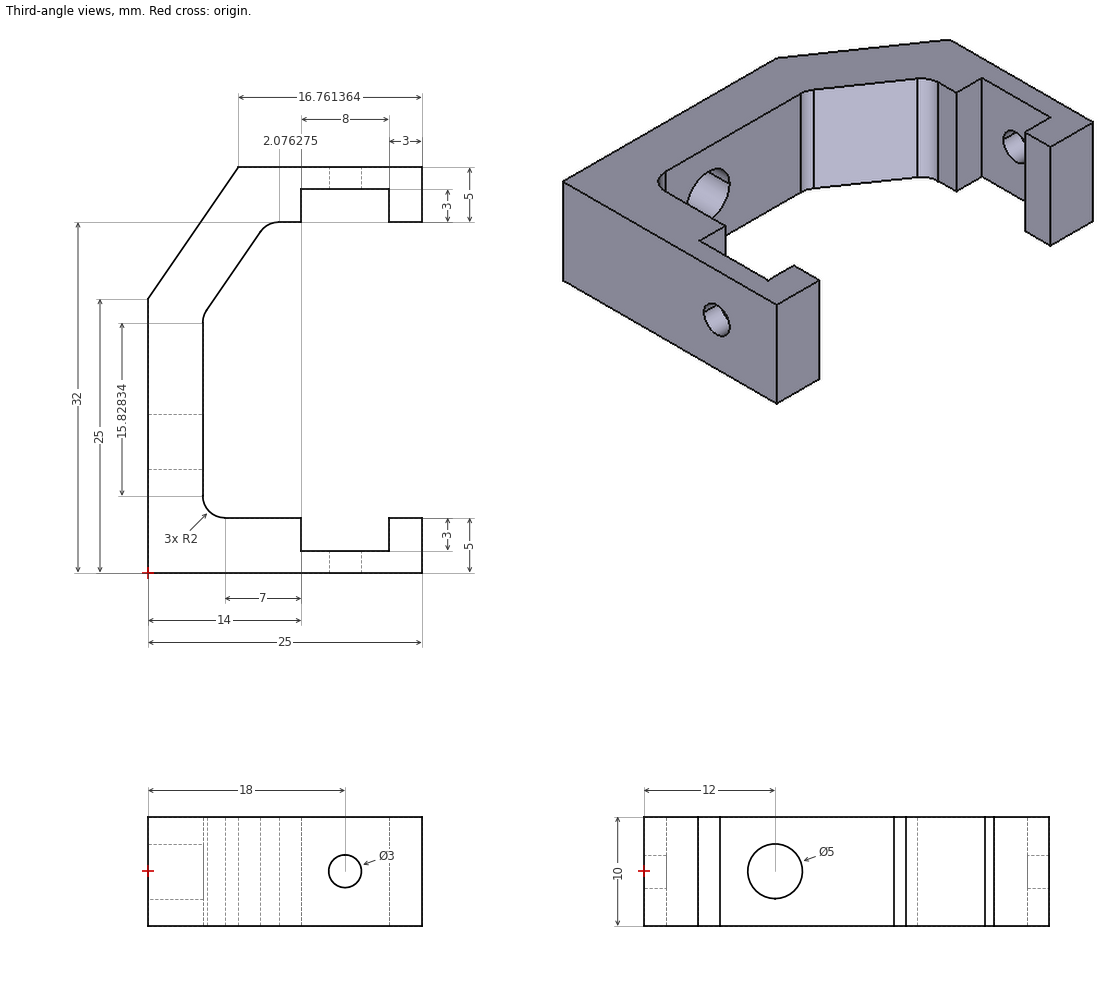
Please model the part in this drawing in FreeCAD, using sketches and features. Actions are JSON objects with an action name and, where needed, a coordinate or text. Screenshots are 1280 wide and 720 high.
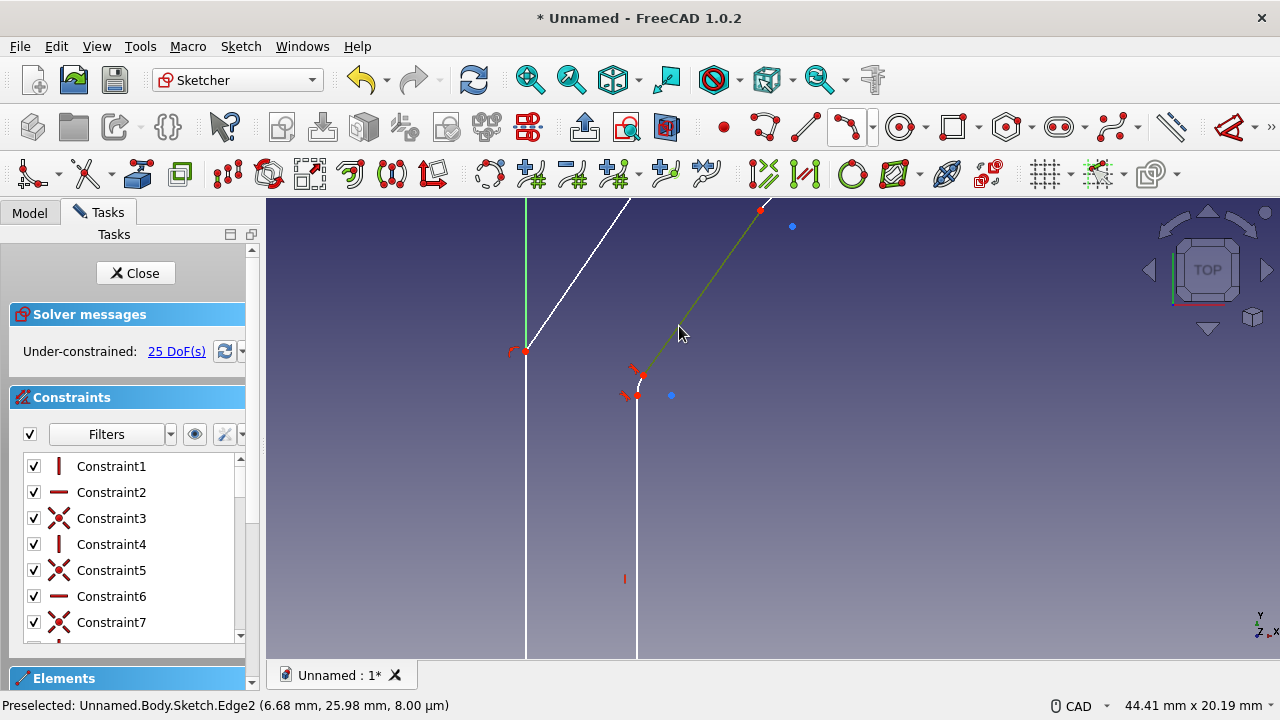
{"action": "scroll", "coordinate": [642, 388], "scroll_direction": "down", "scroll_amount": 5}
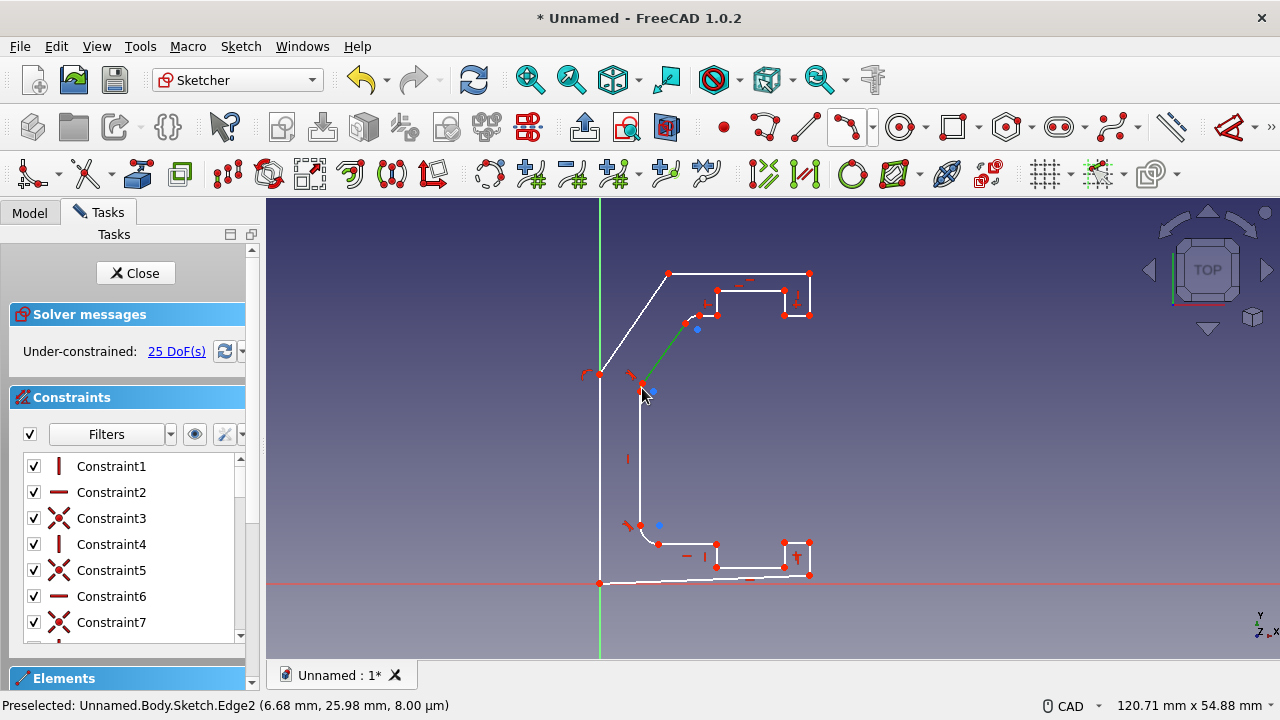
{"action": "scroll", "coordinate": [695, 316], "scroll_direction": "up", "scroll_amount": 6}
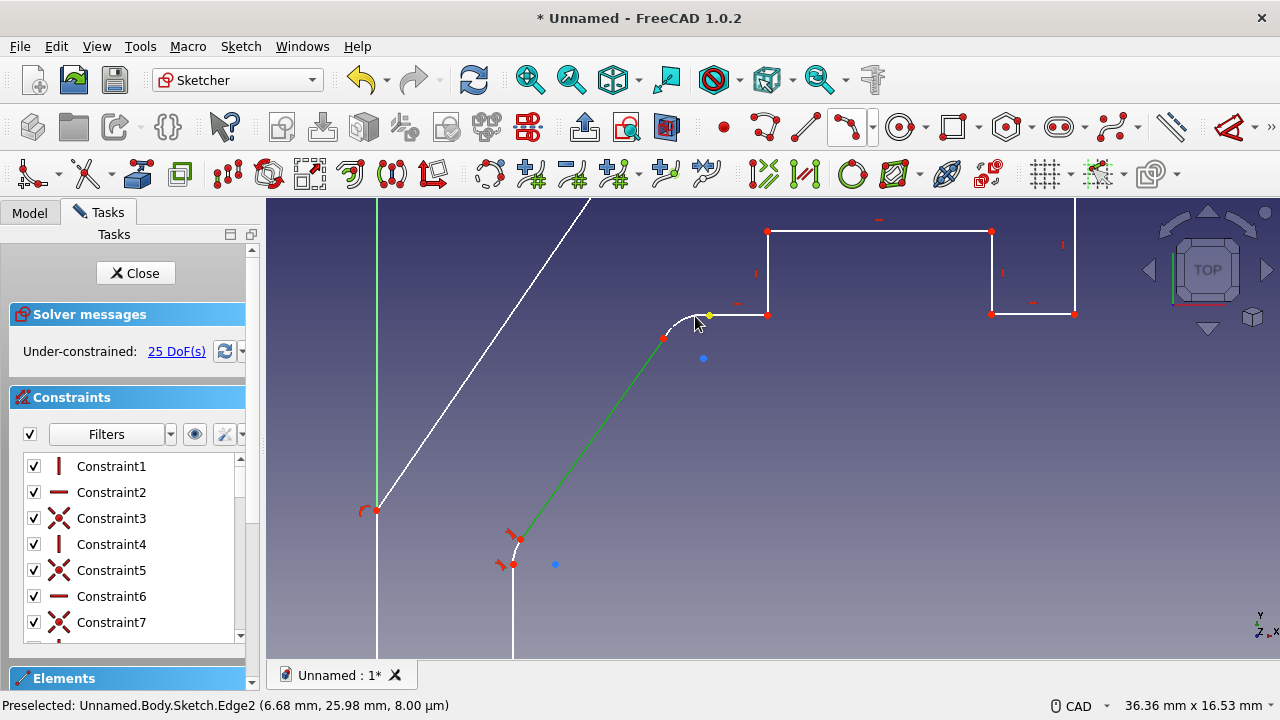
{"action": "left_click", "coordinate": [693, 316]}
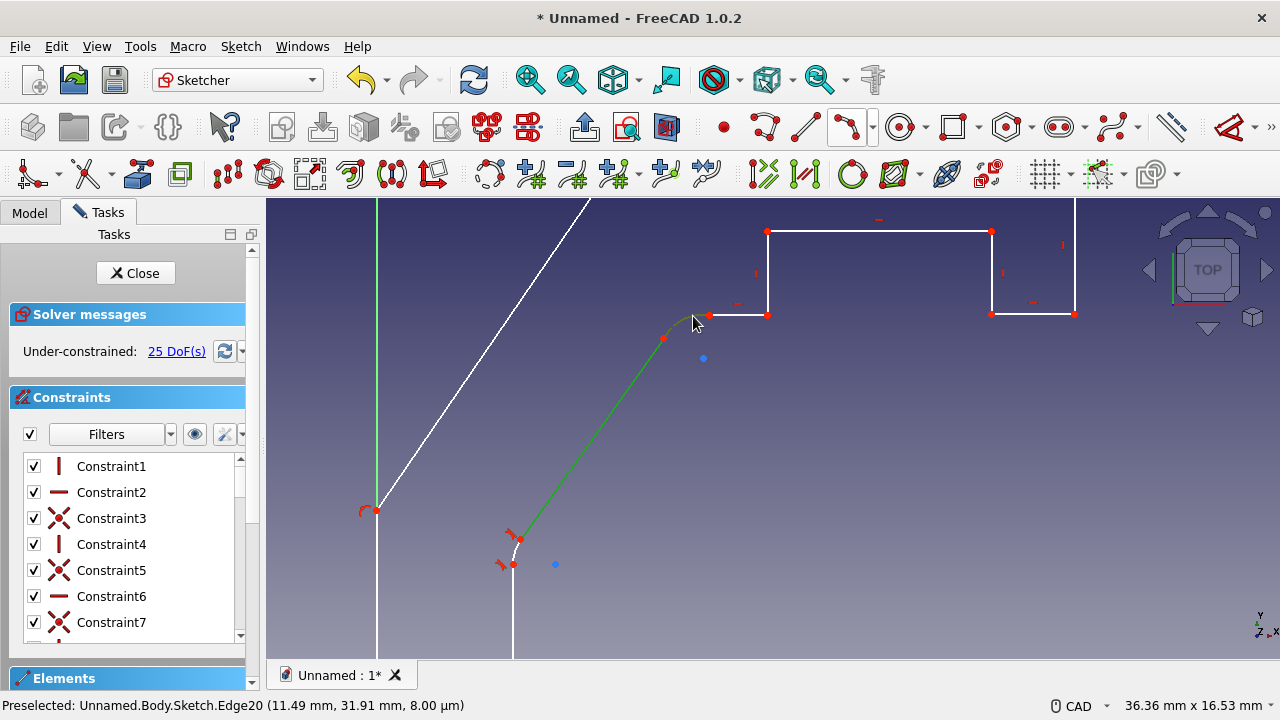
{"action": "key", "text": "t"}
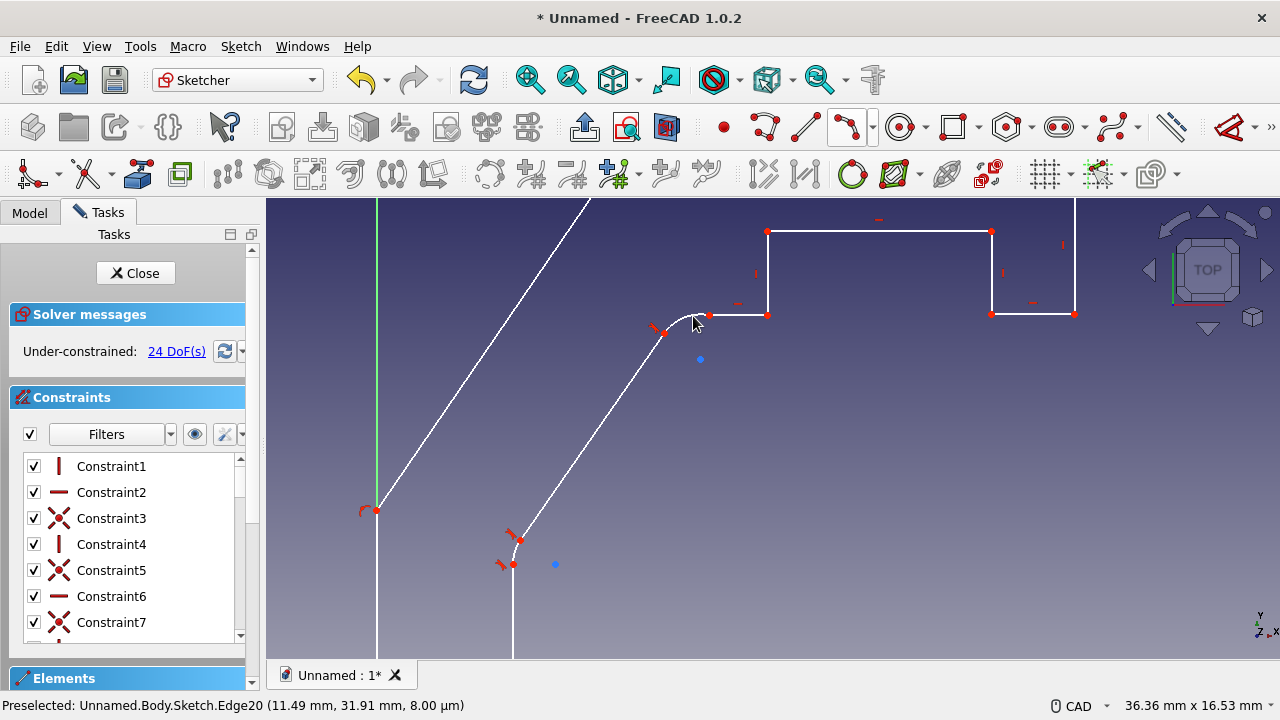
{"action": "left_click", "coordinate": [727, 315]}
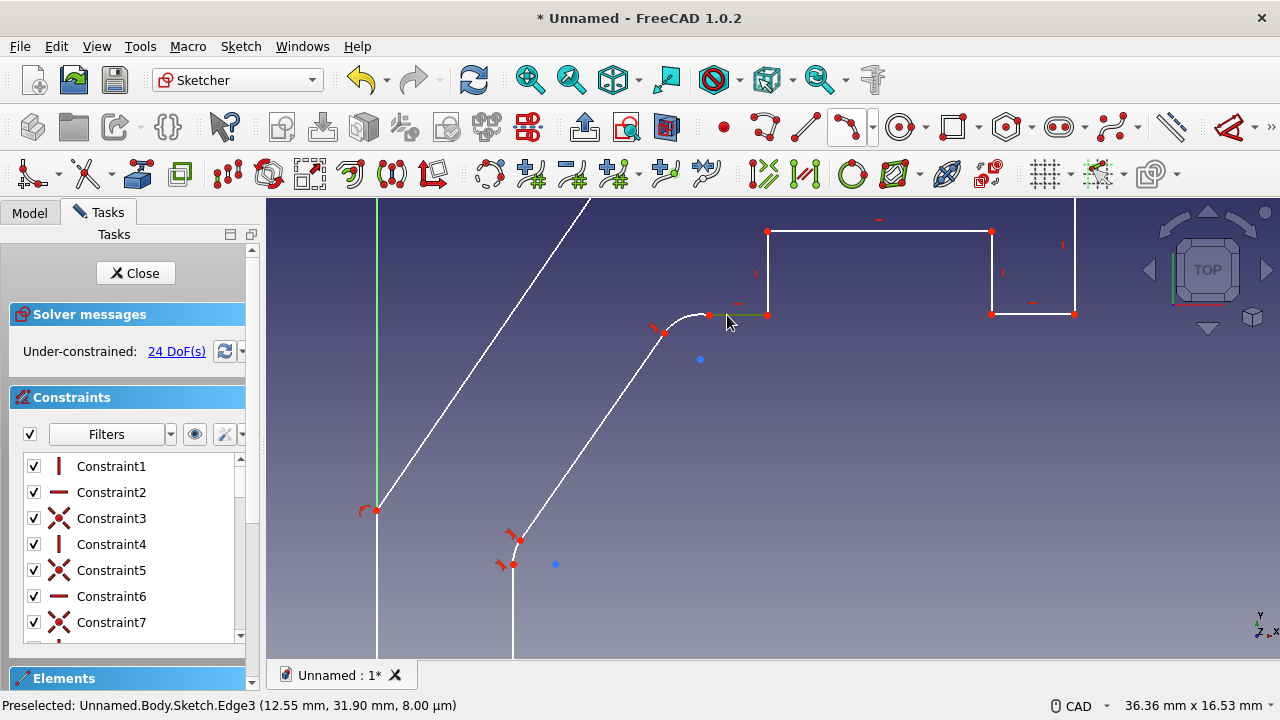
{"action": "left_click", "coordinate": [694, 315]}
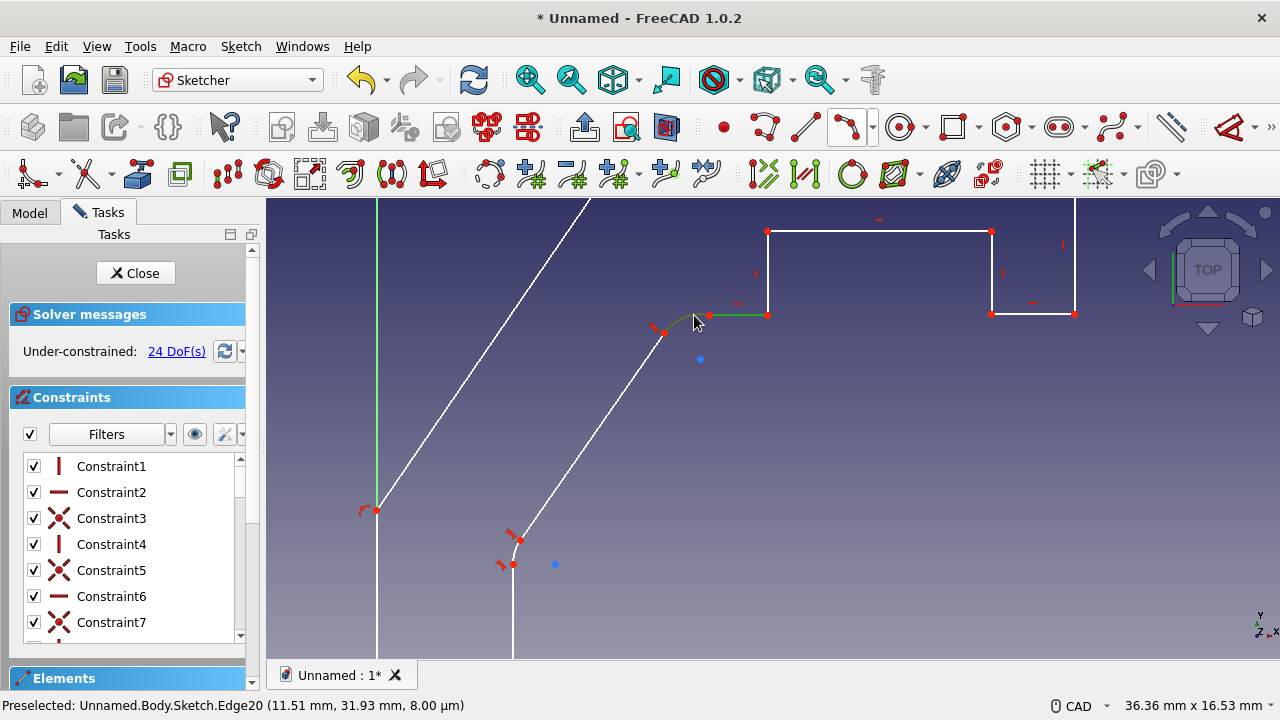
{"action": "key", "text": "t"}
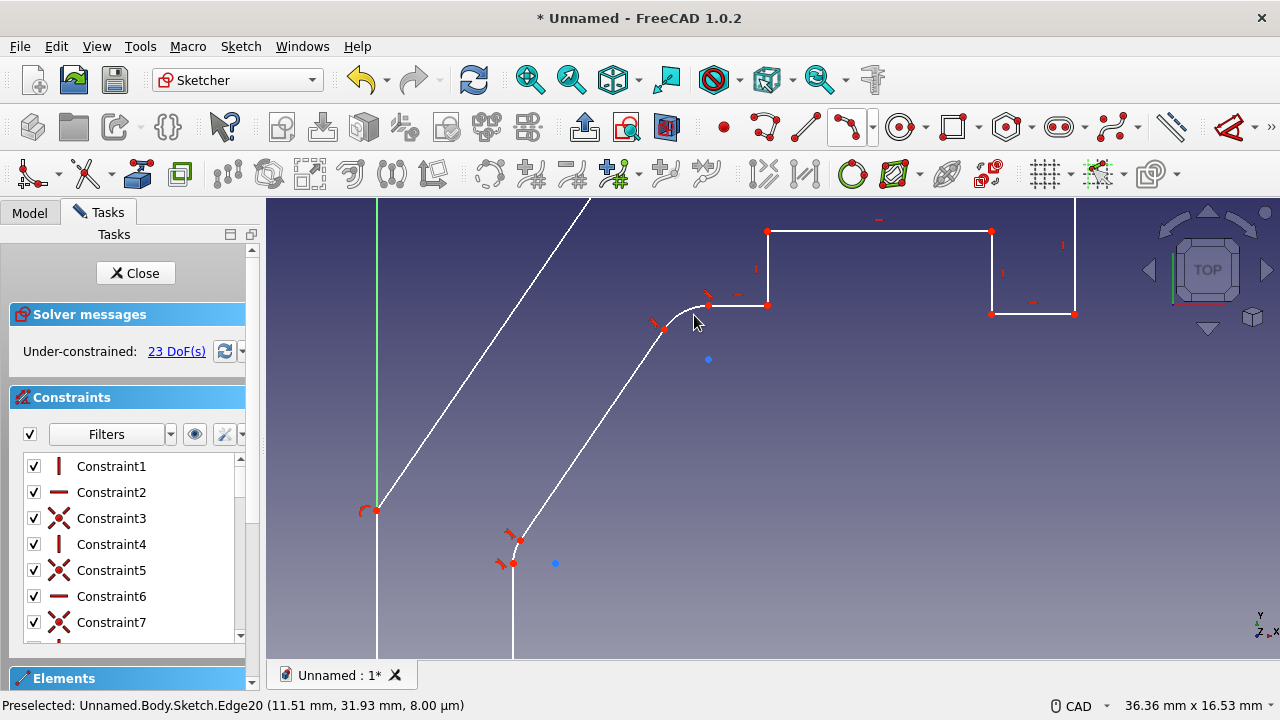
{"action": "scroll", "coordinate": [695, 316], "scroll_direction": "down", "scroll_amount": 6}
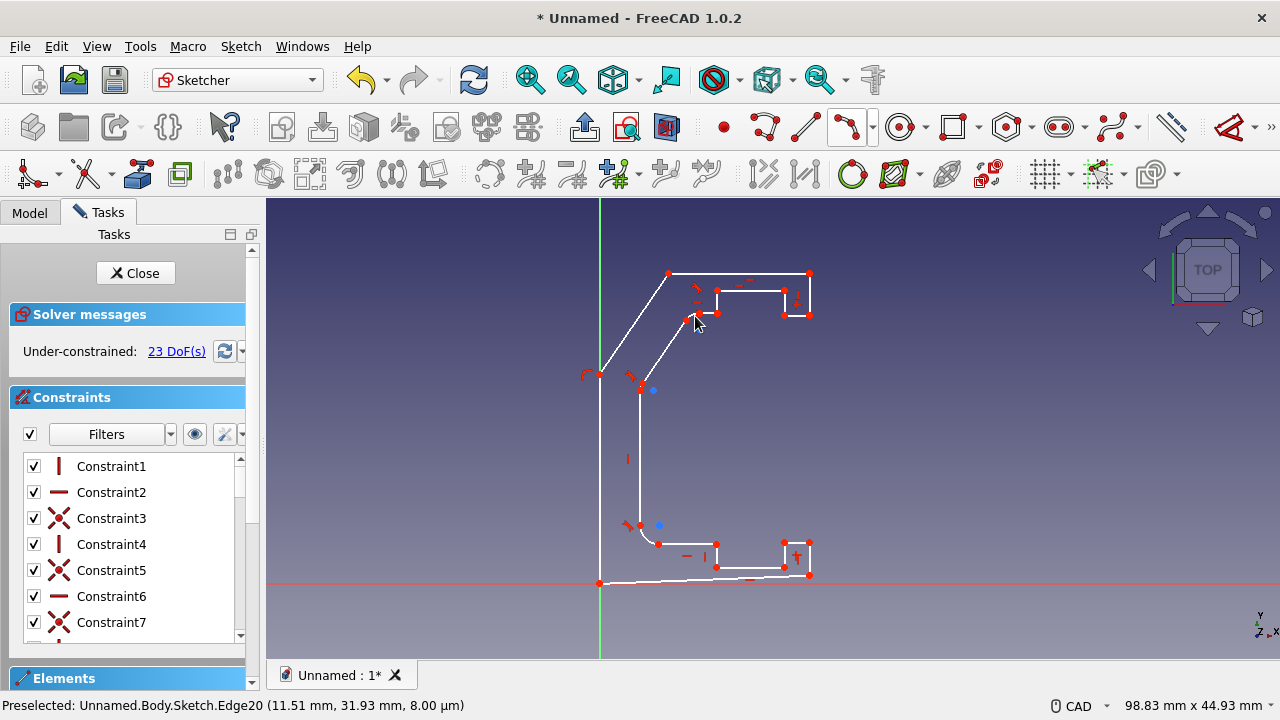
{"action": "left_click", "coordinate": [699, 544]}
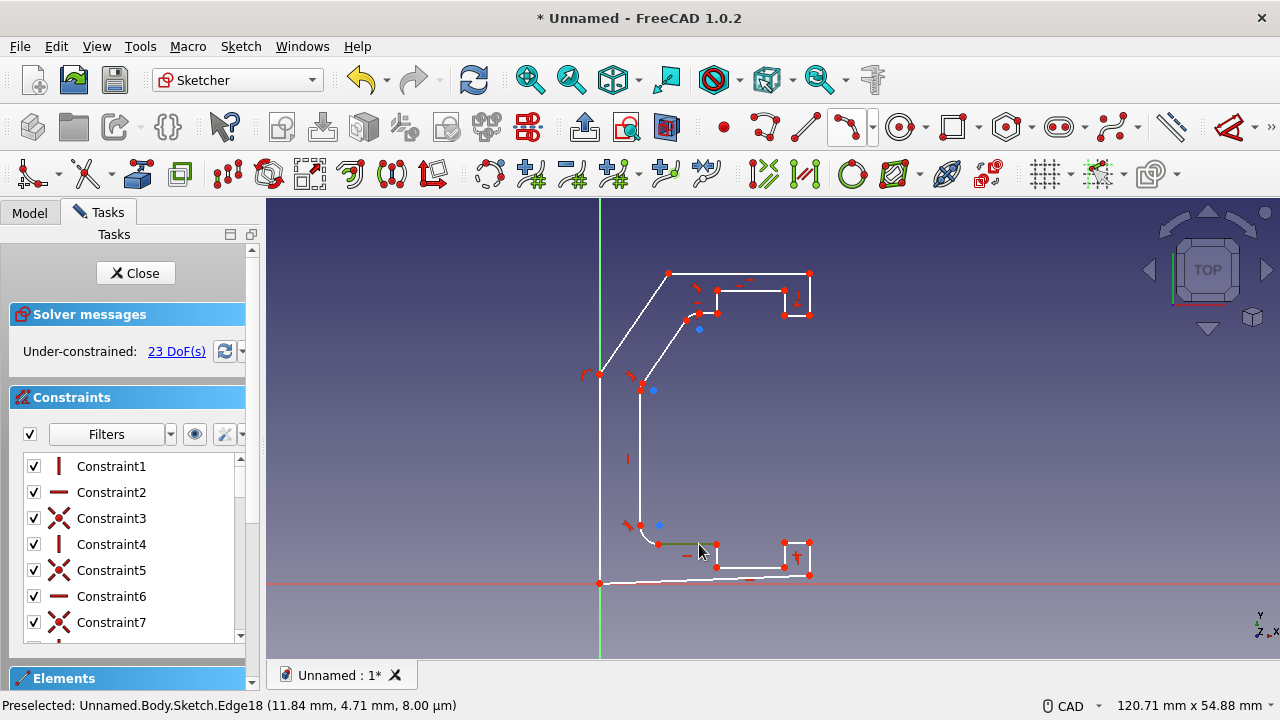
{"action": "left_click", "coordinate": [646, 539]}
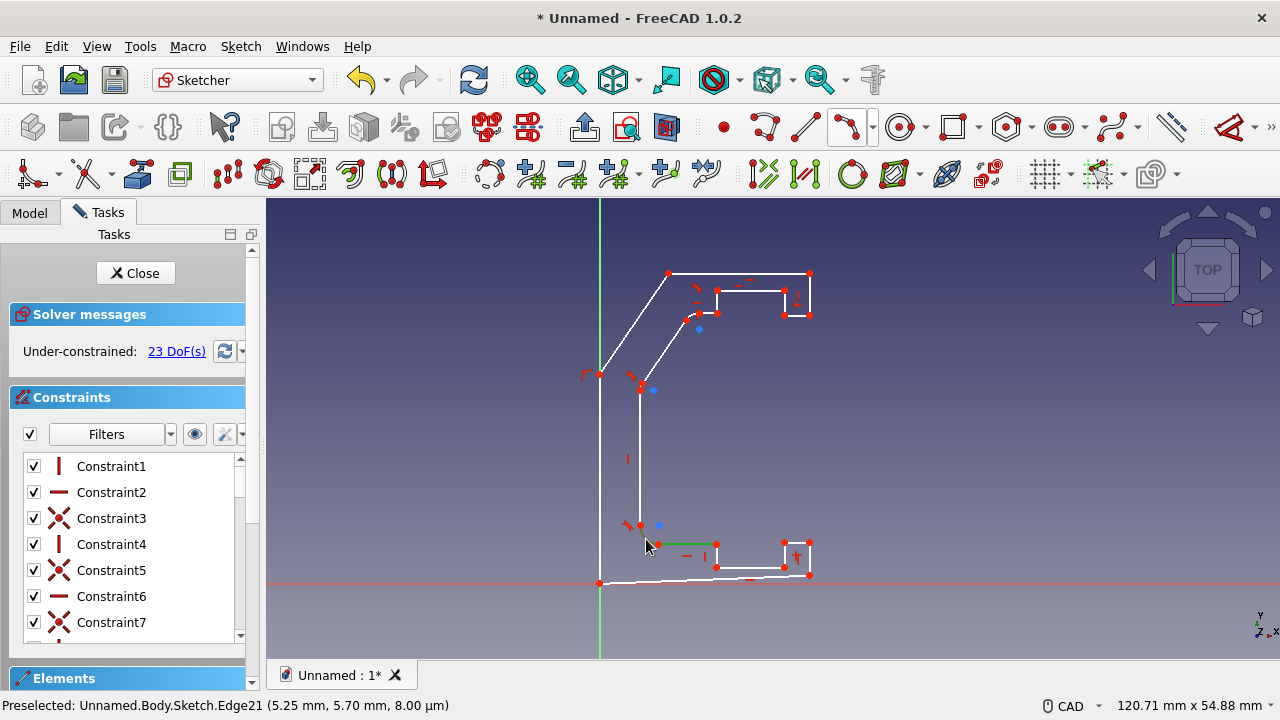
{"action": "key", "text": "t"}